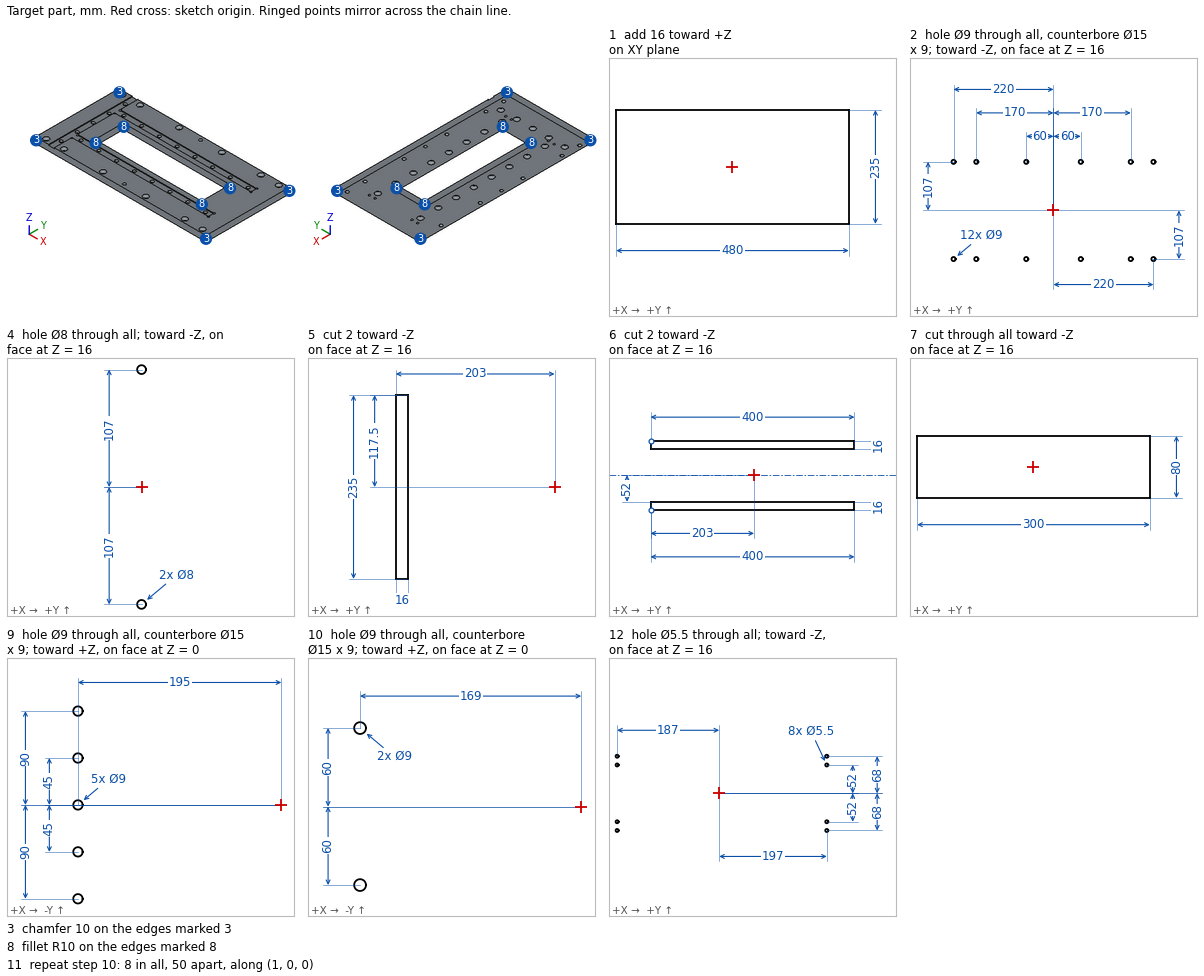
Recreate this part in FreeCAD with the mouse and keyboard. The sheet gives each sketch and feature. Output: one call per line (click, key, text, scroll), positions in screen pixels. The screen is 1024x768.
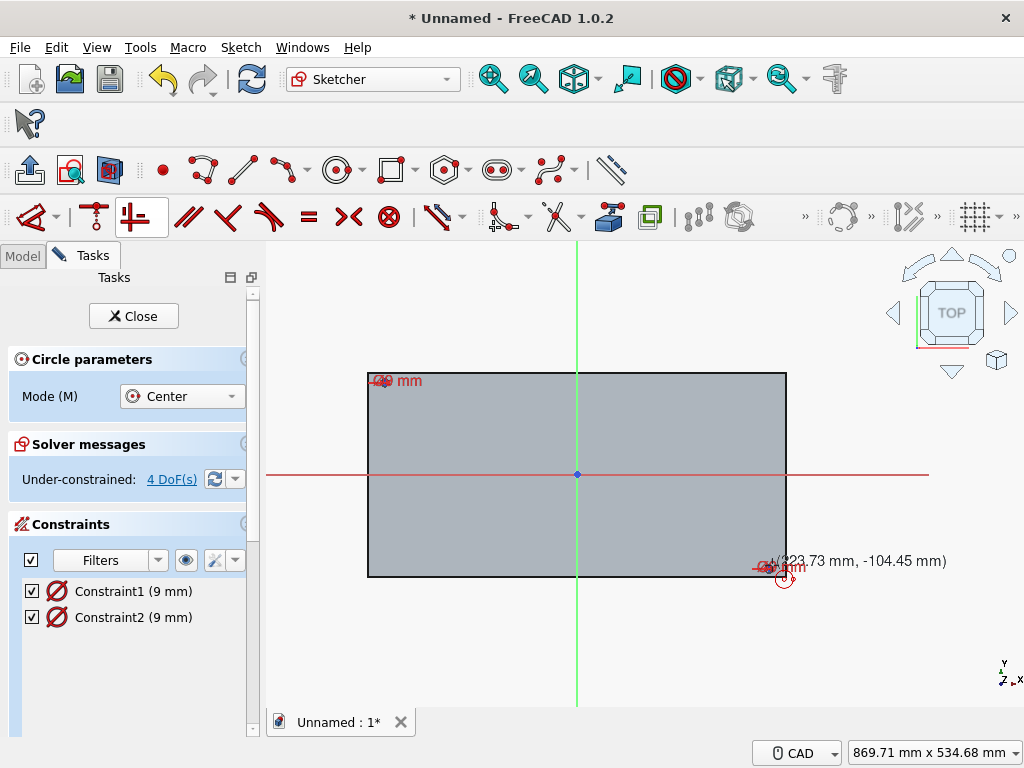
scroll(385, 568, up, 9)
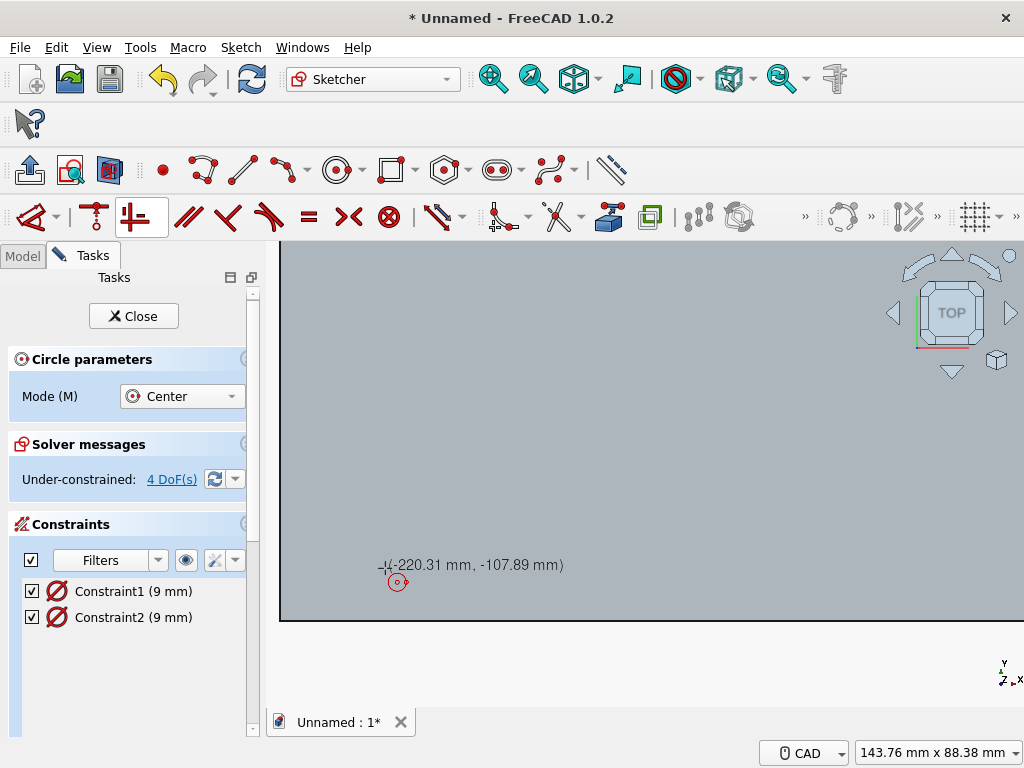
scroll(385, 568, down, 9)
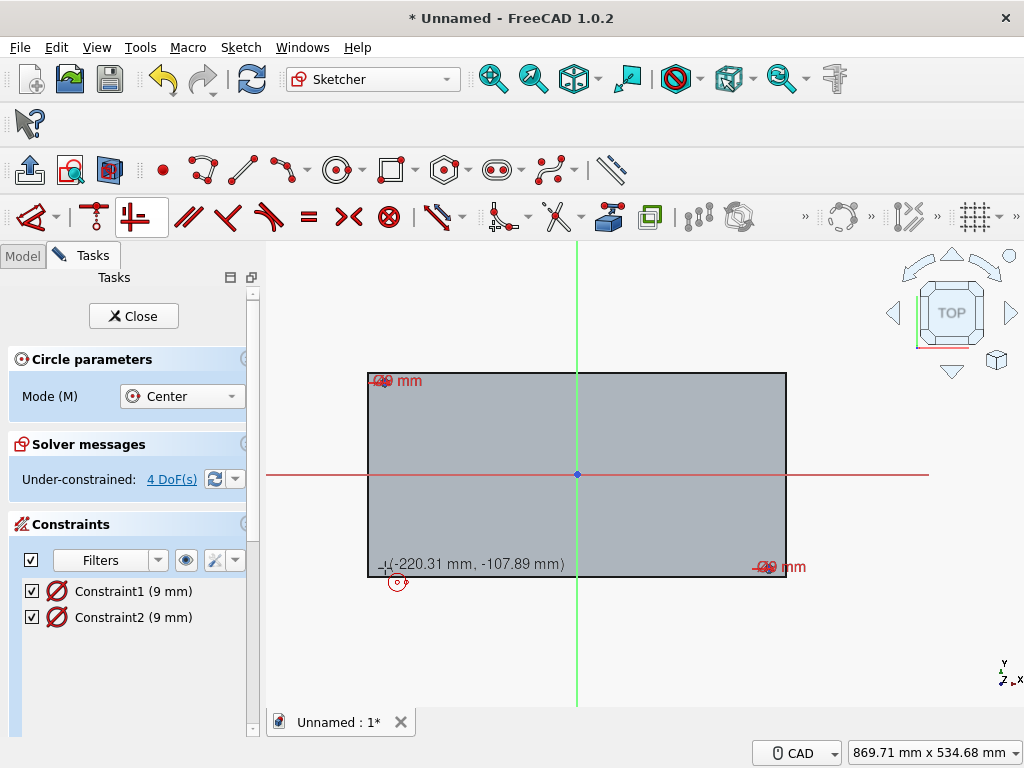
click(385, 568)
move(388, 565)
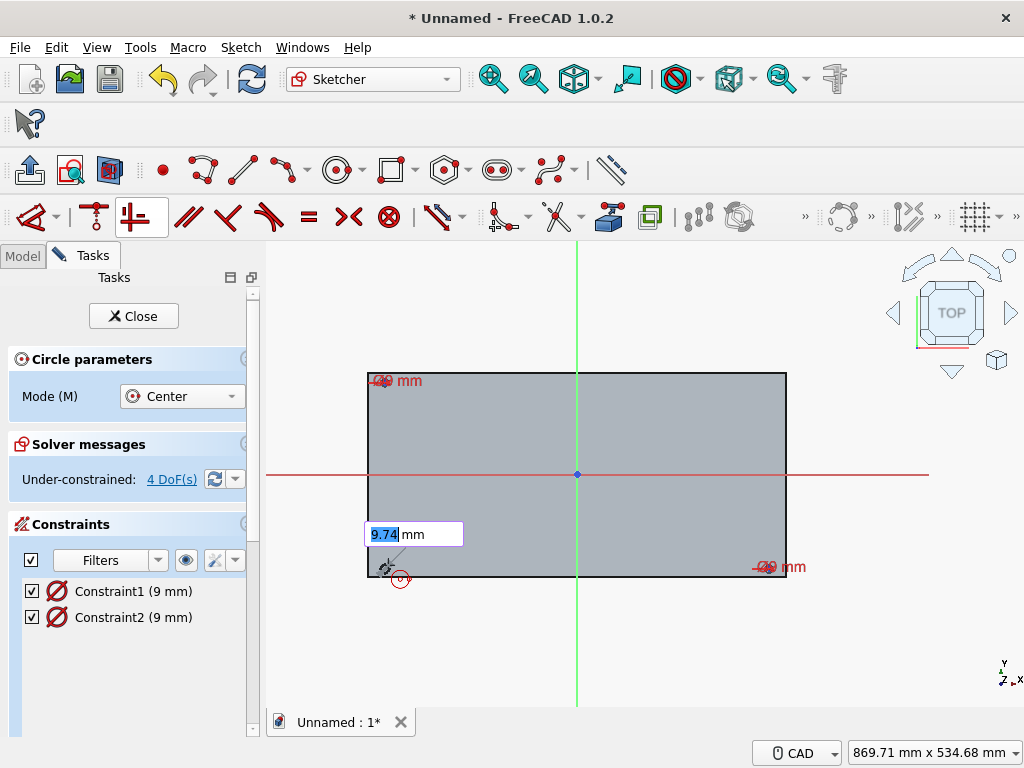
text(9)
key(Return)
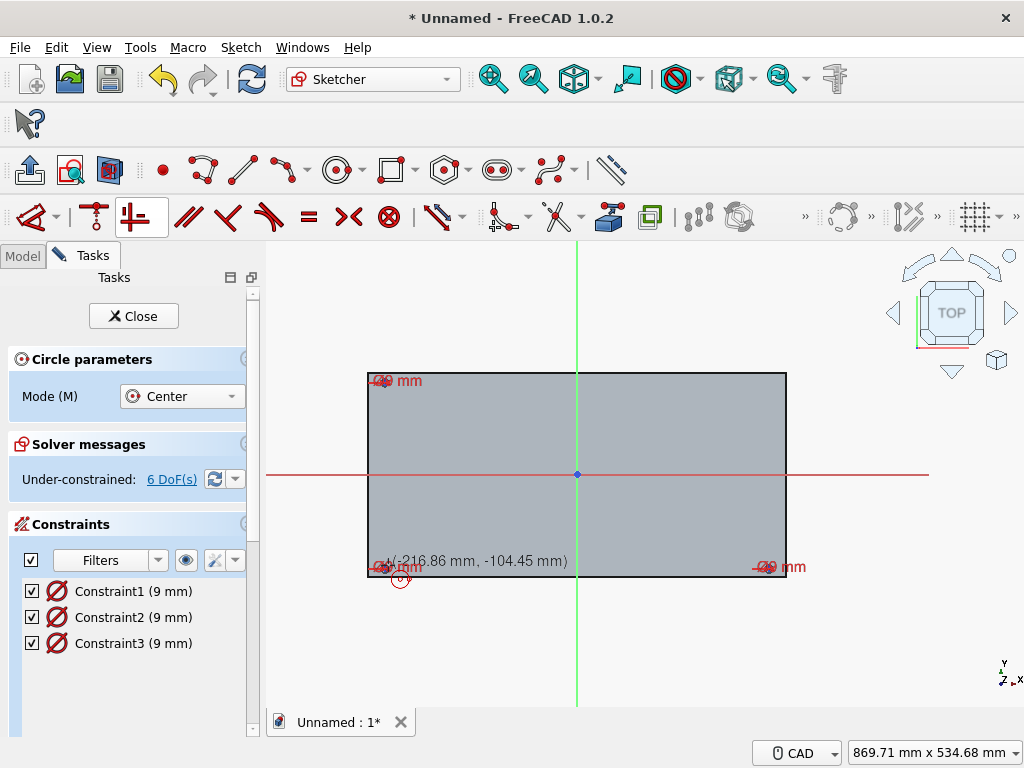
scroll(769, 382, up, 9)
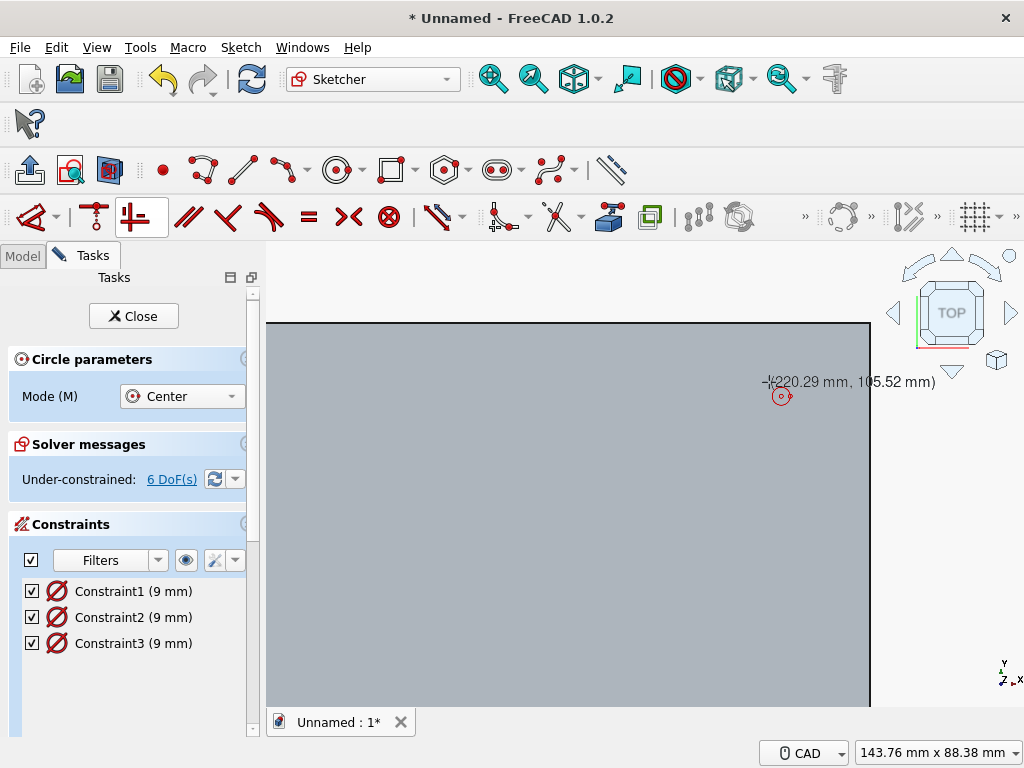
scroll(769, 381, down, 9)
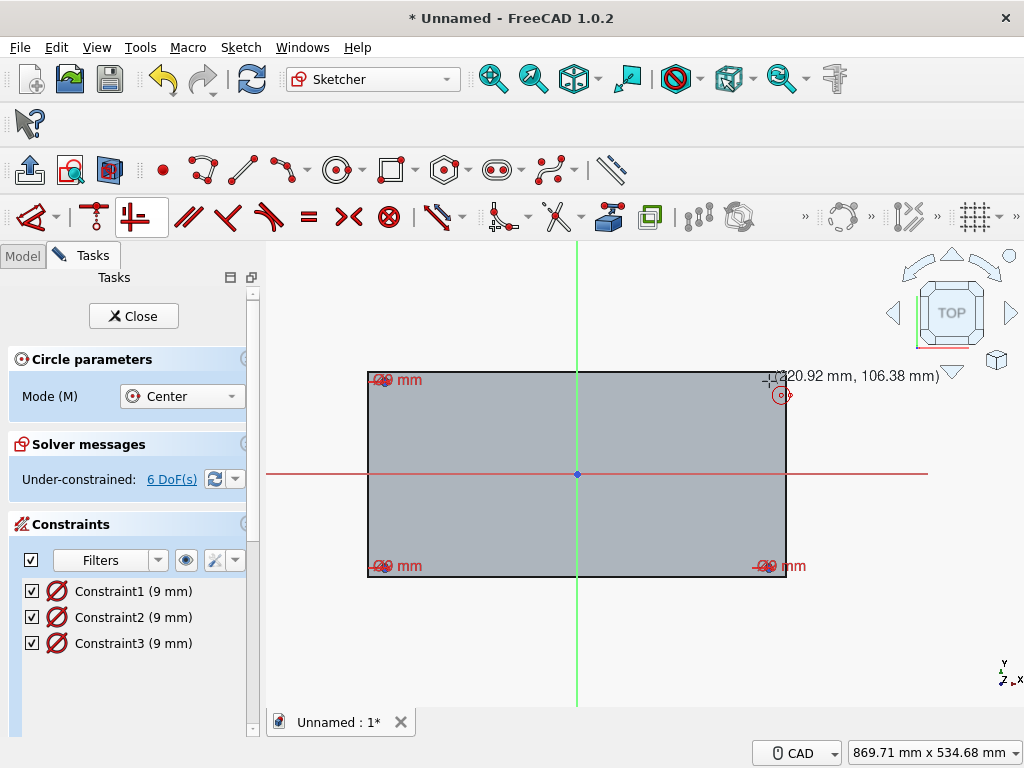
click(769, 381)
move(772, 378)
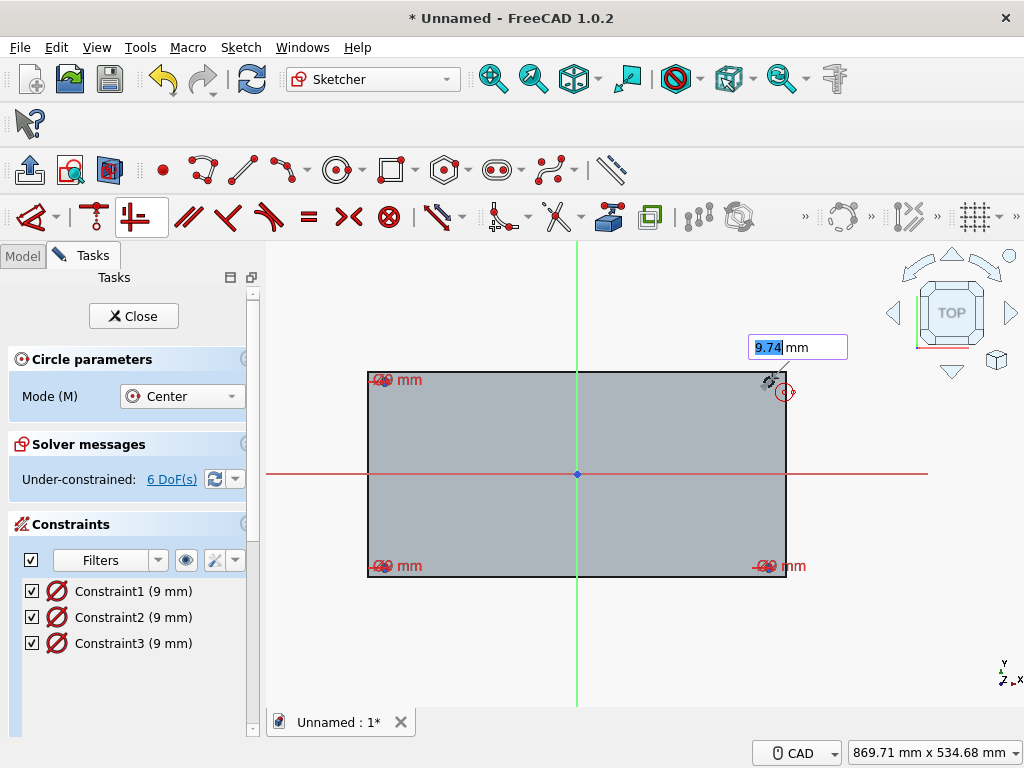
text(9)
key(Return)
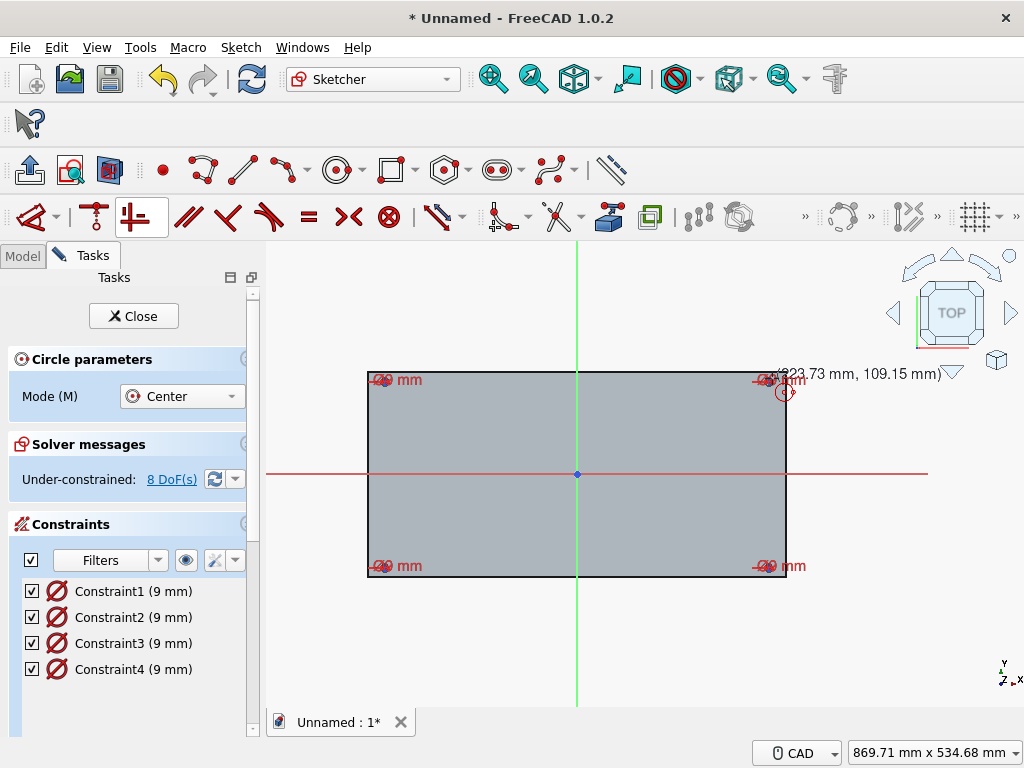
scroll(429, 381, up, 9)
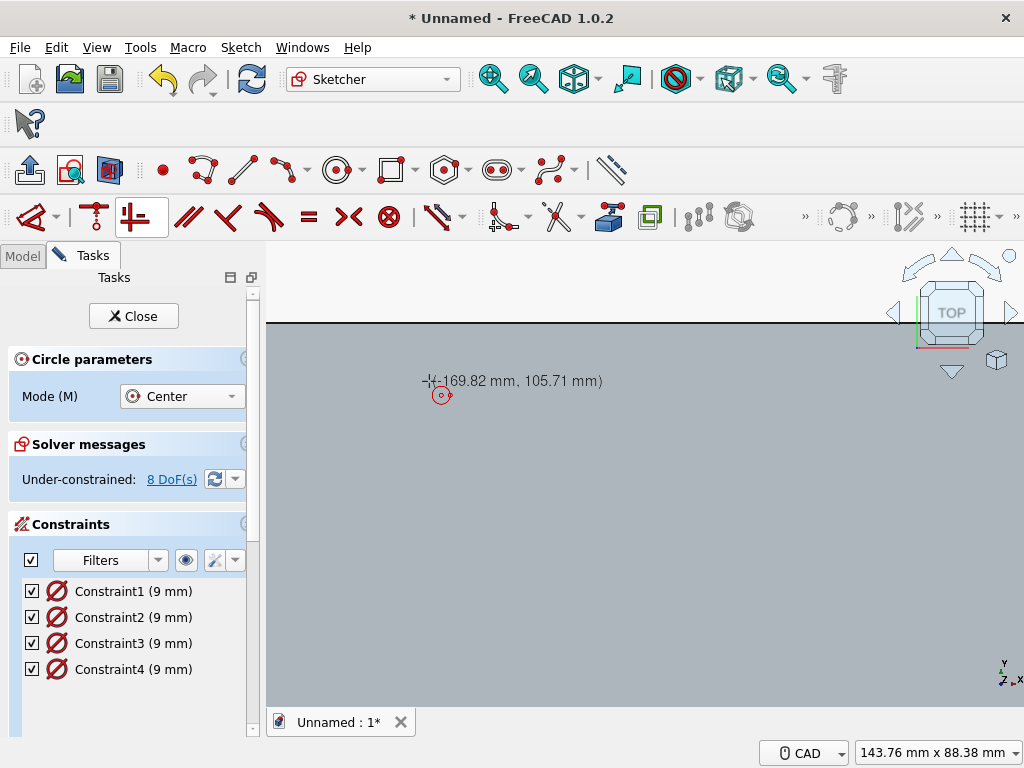
scroll(429, 381, down, 9)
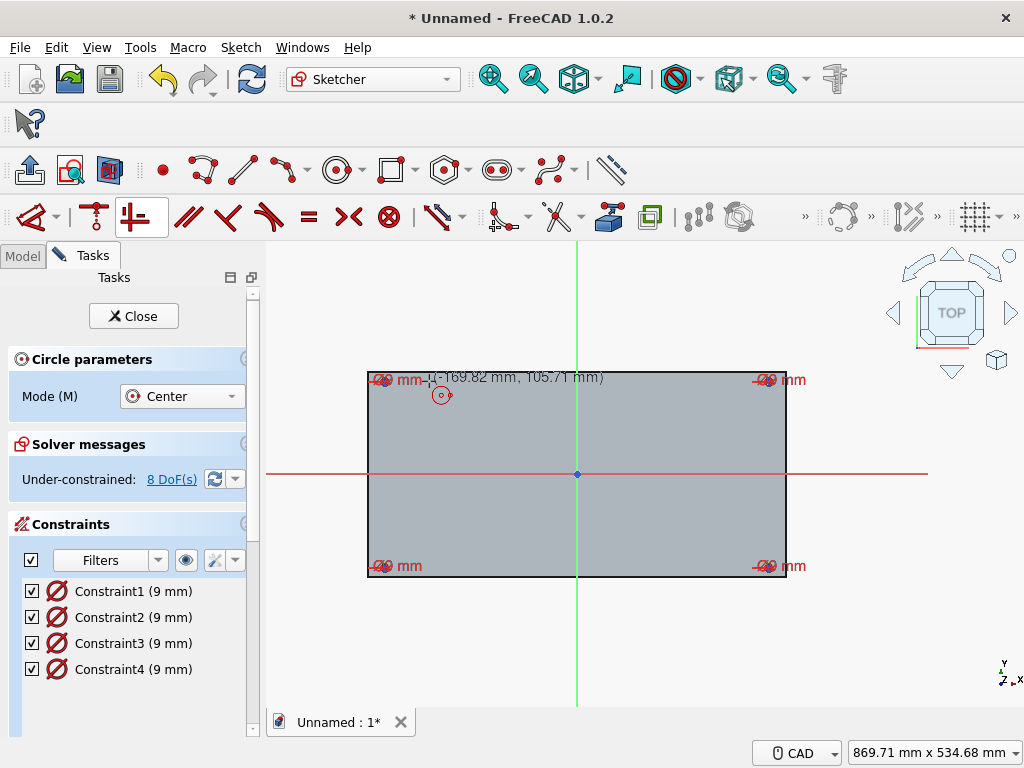
click(429, 381)
move(432, 378)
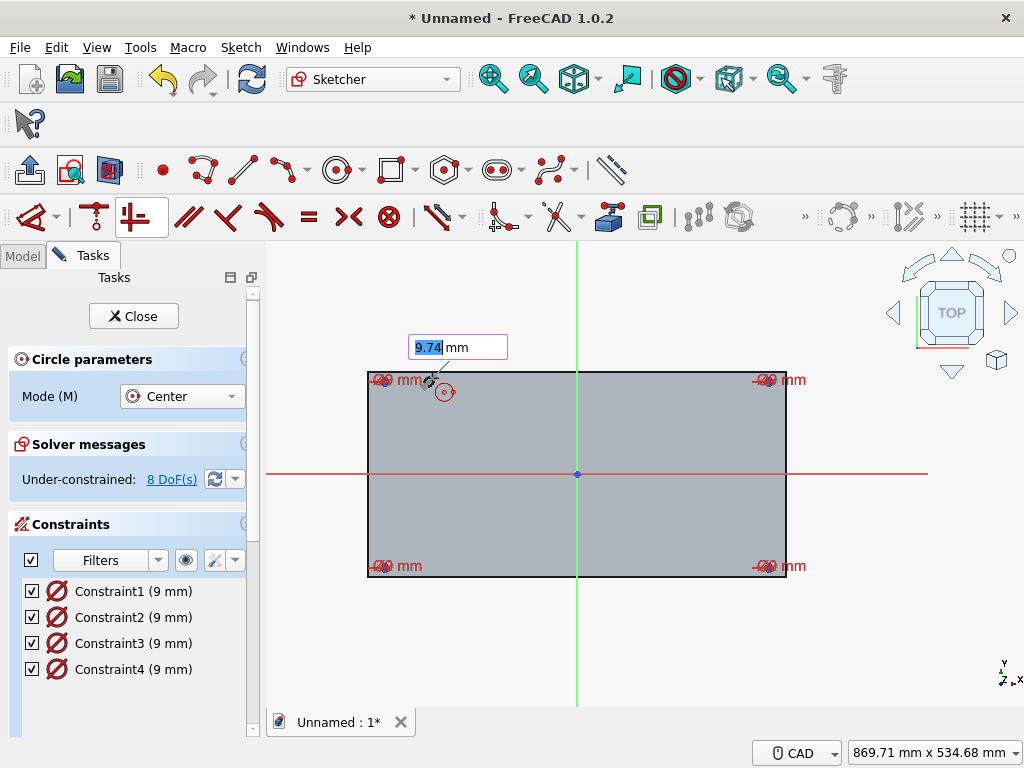
text(9)
key(Return)